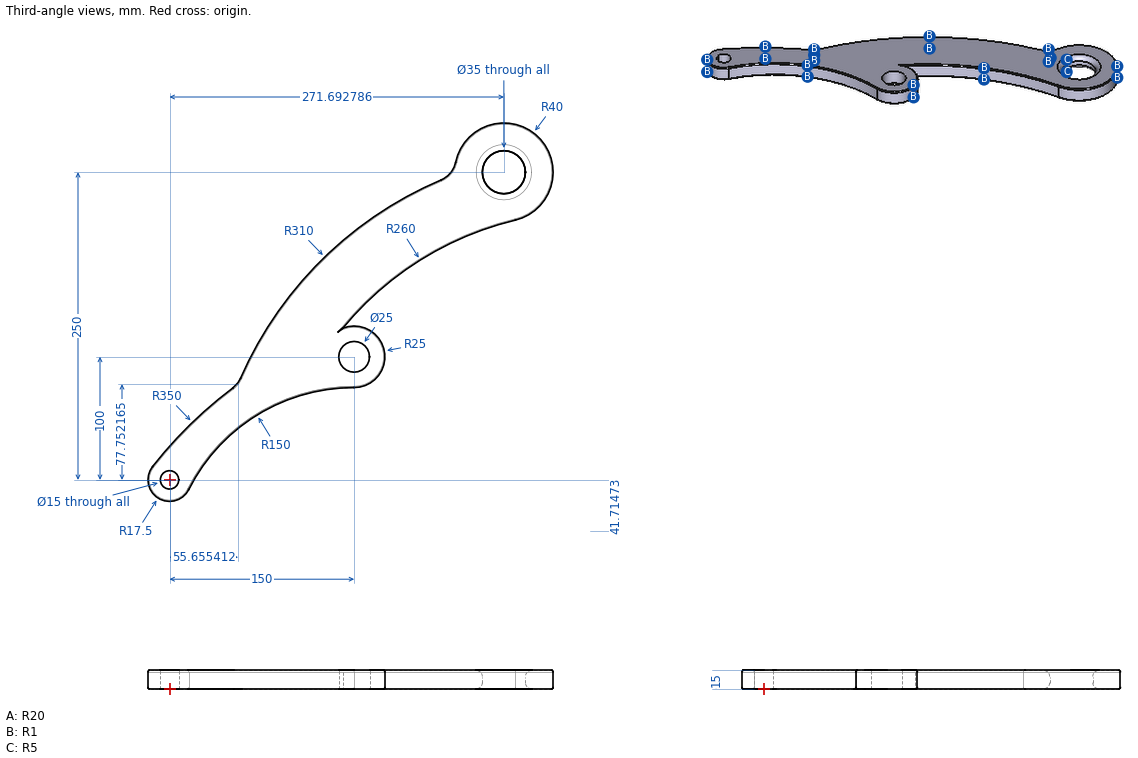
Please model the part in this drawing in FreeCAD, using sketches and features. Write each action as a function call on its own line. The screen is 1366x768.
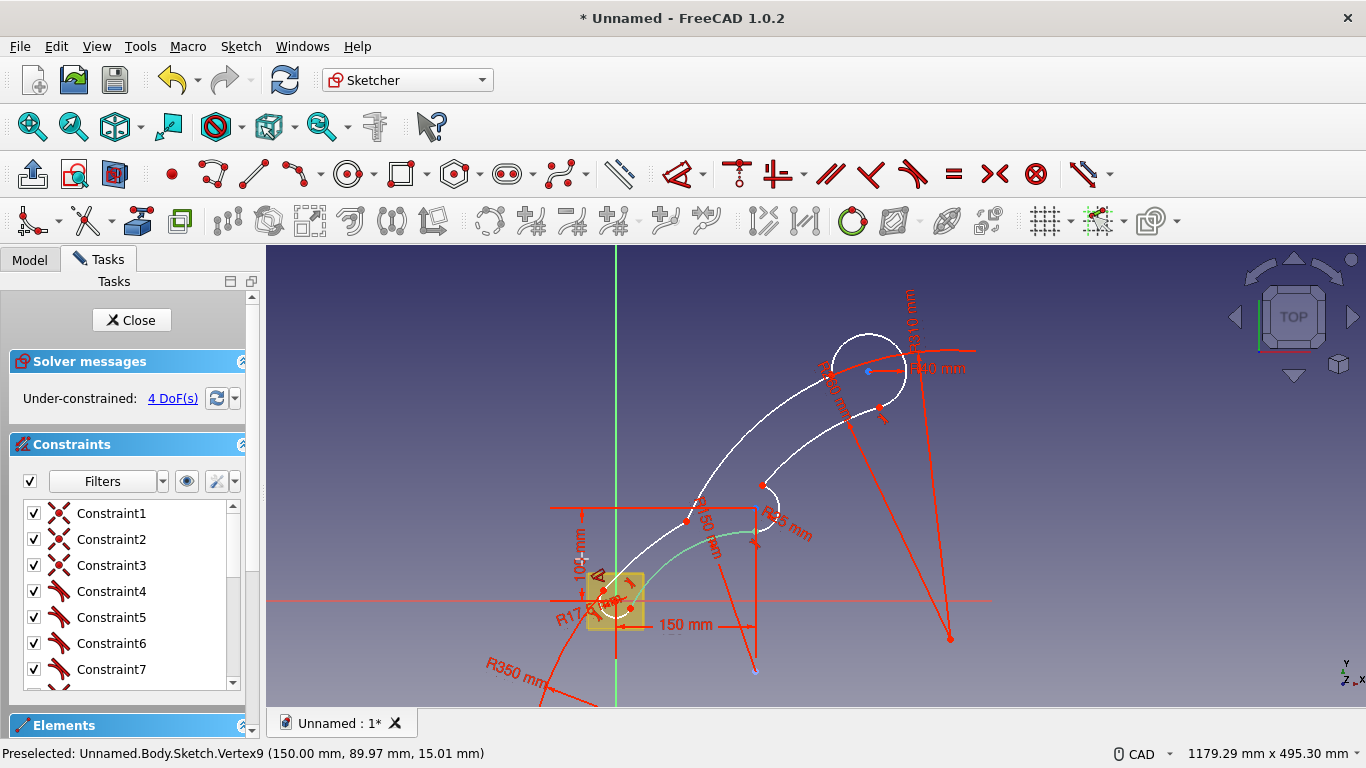
click(869, 372)
click(582, 486)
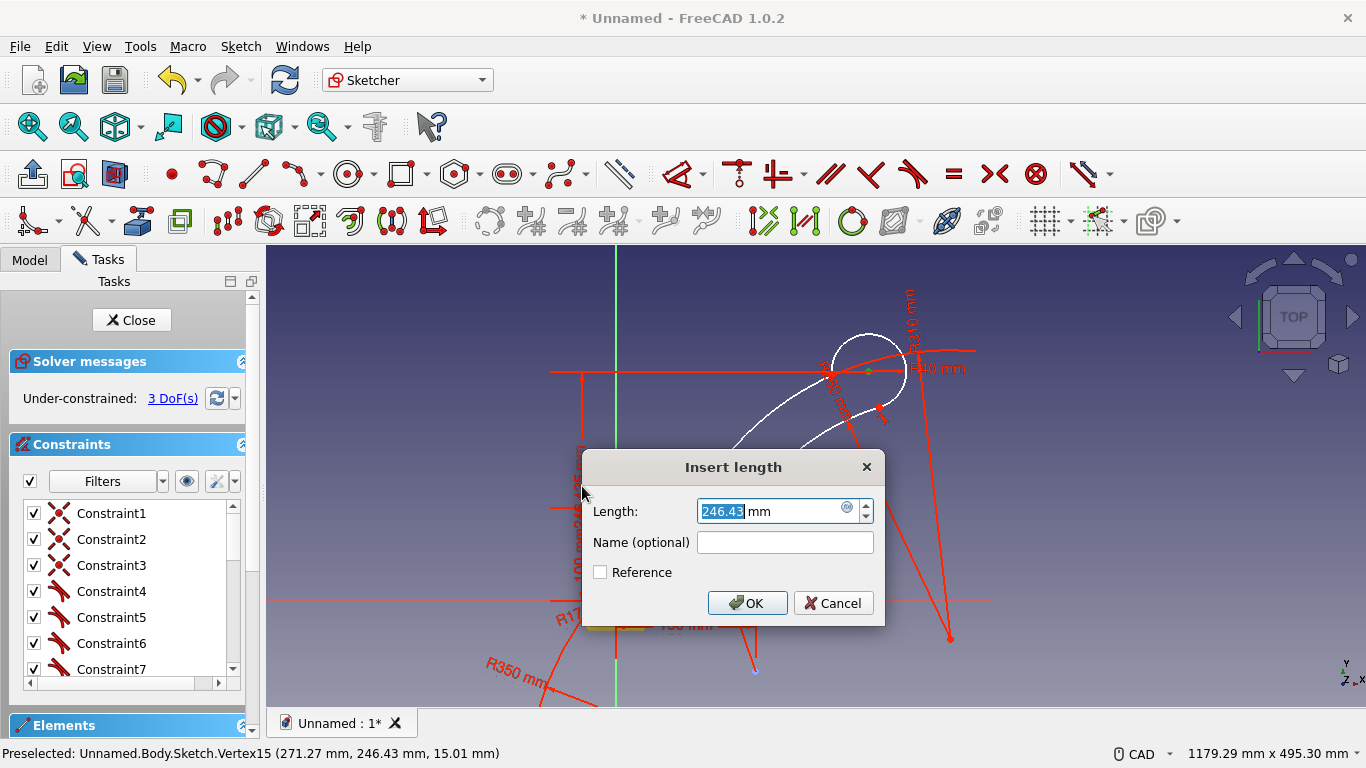
text(250)
key(Return)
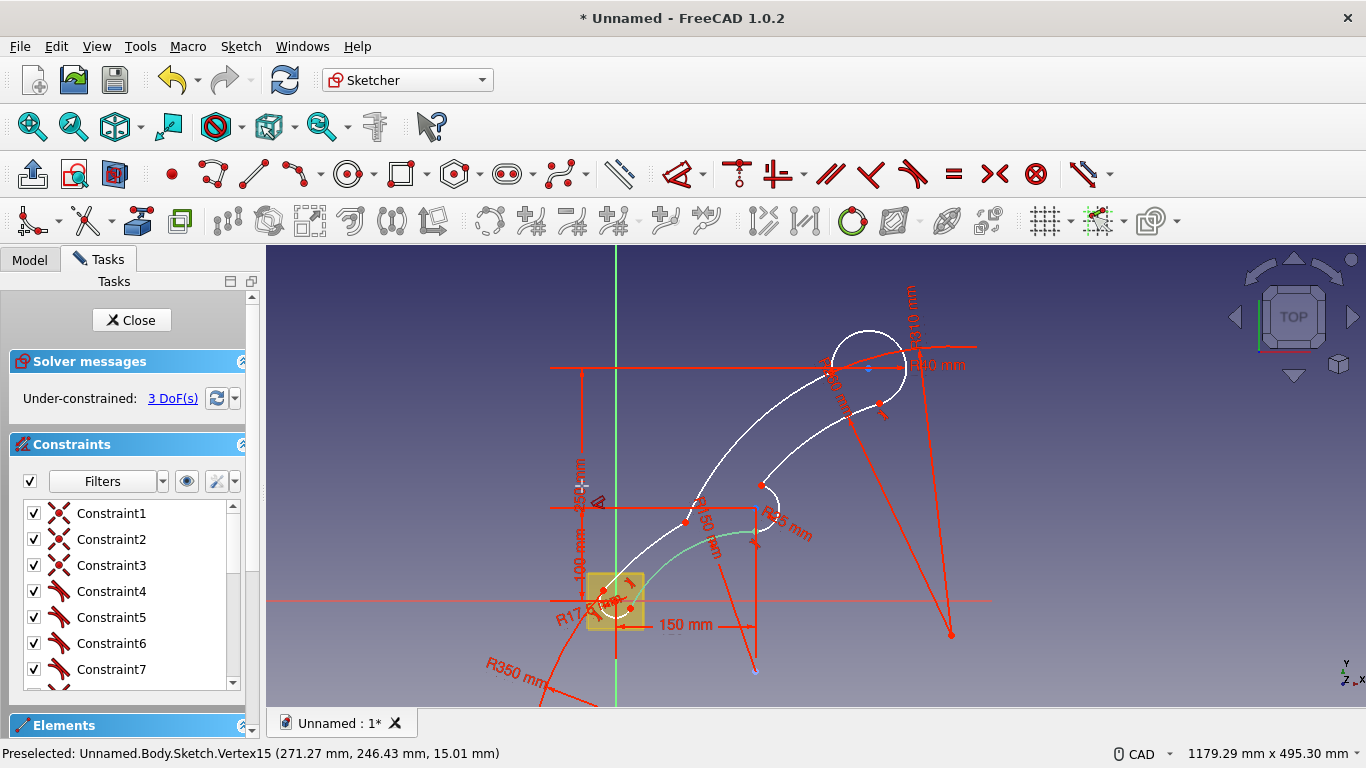
click(952, 636)
click(986, 618)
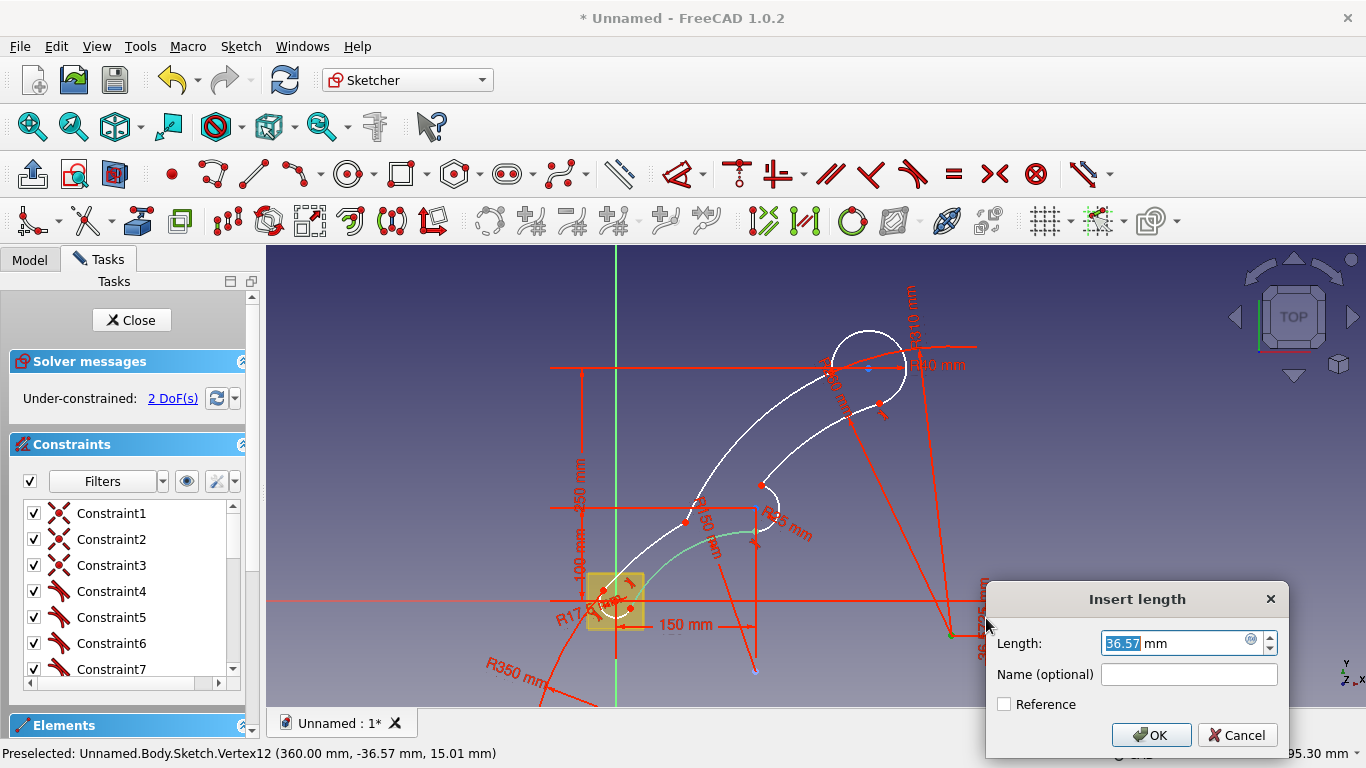
text(41.71473)
key(Return)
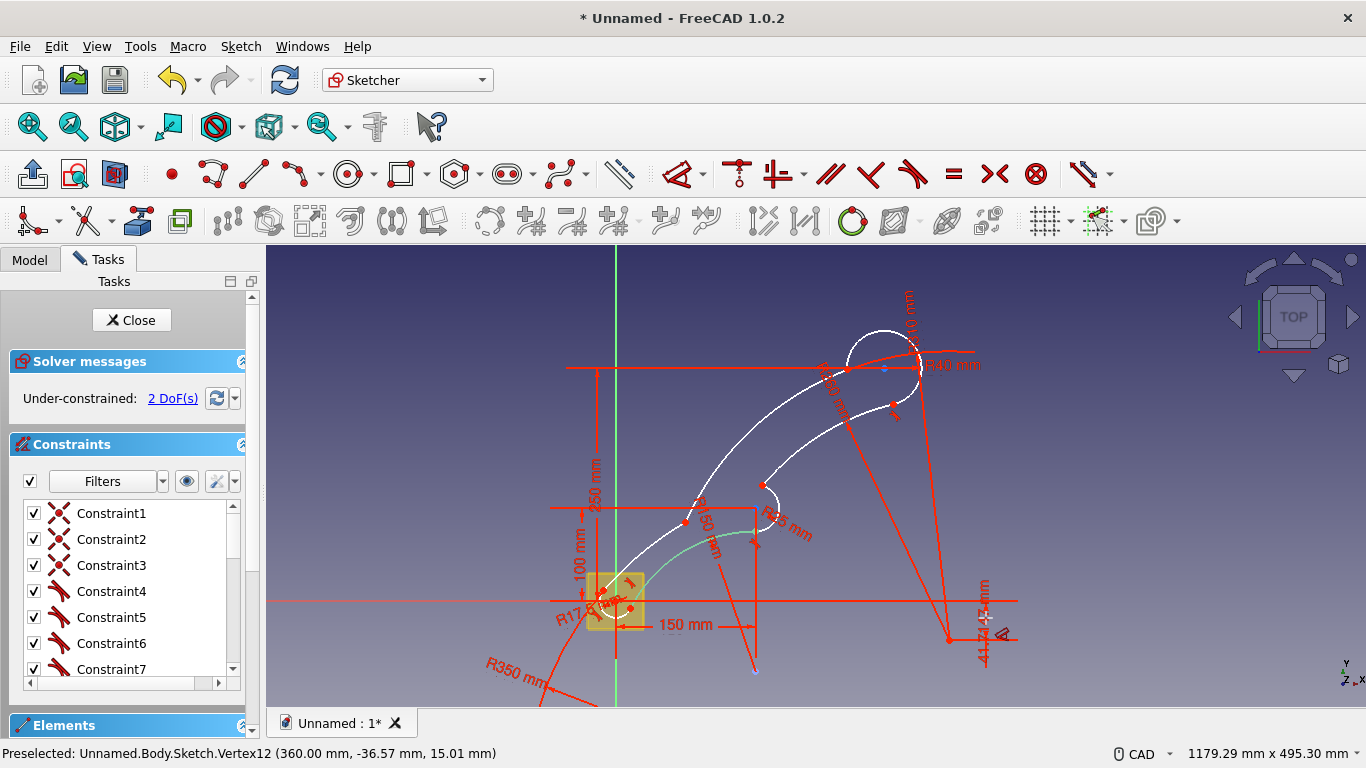
click(686, 522)
click(667, 488)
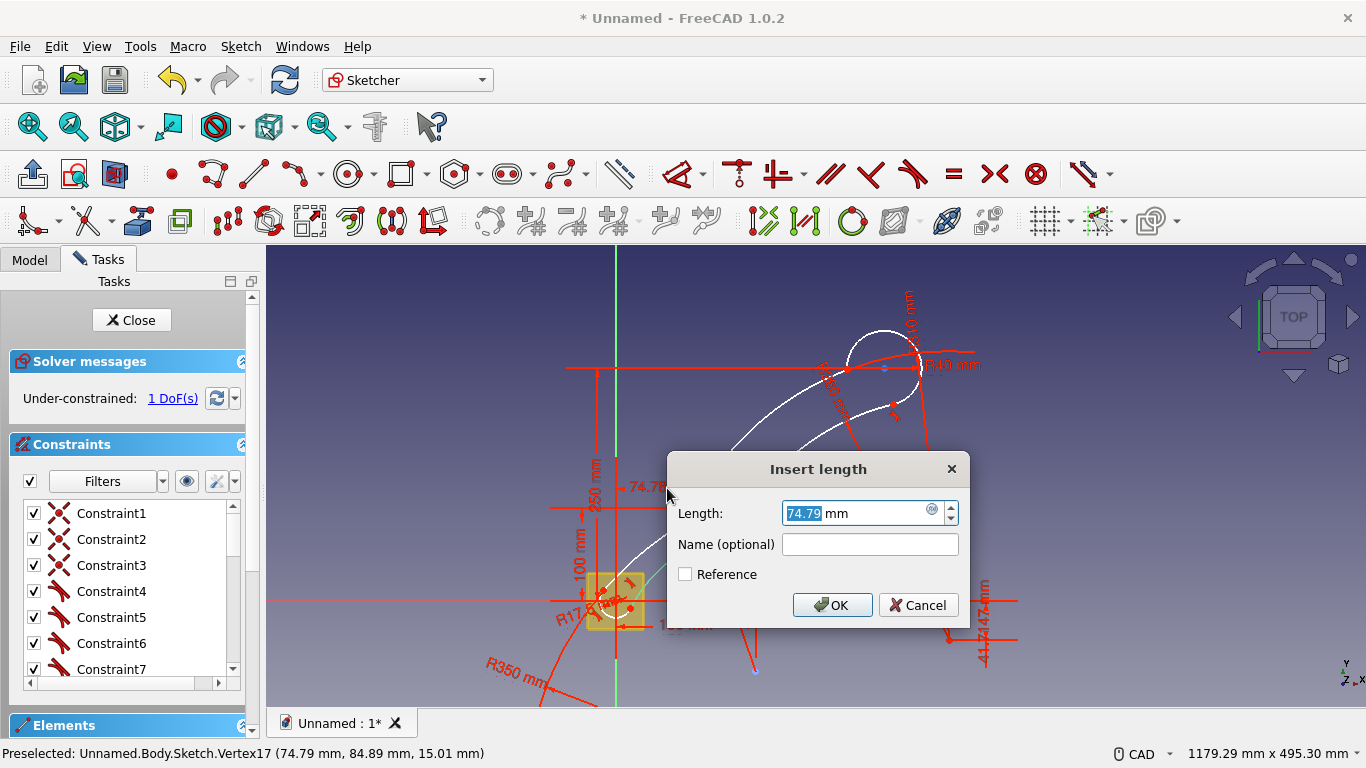
text(55.655412)
key(Return)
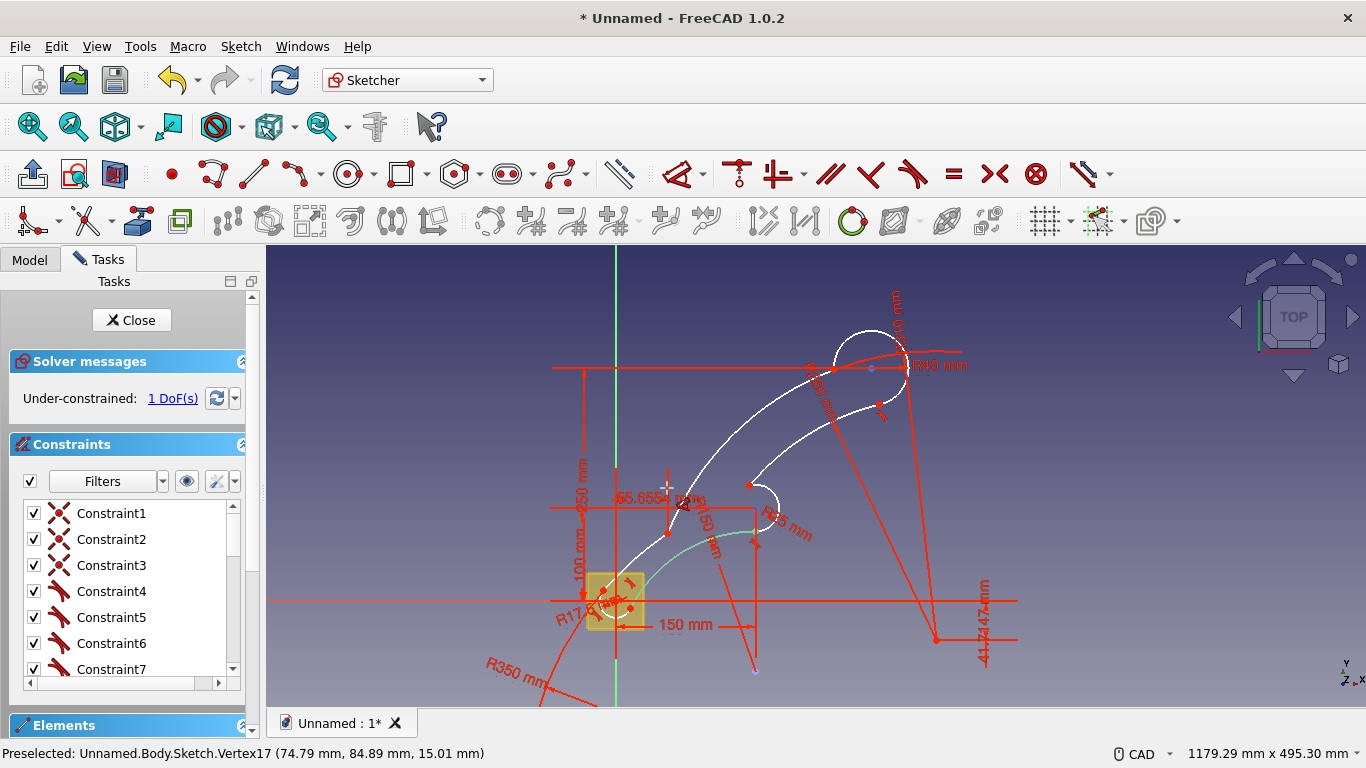
click(668, 533)
click(582, 583)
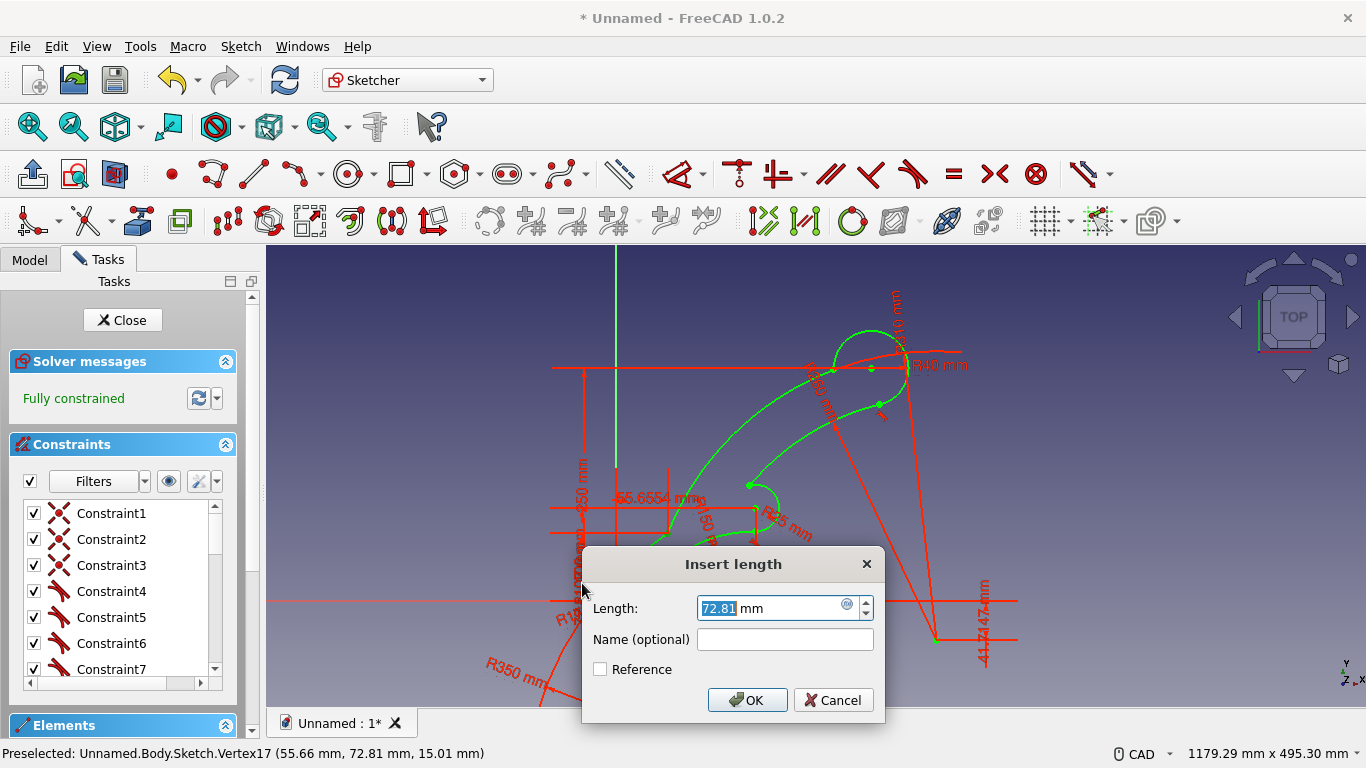
text(77.752165)
key(Return)
key(Escape)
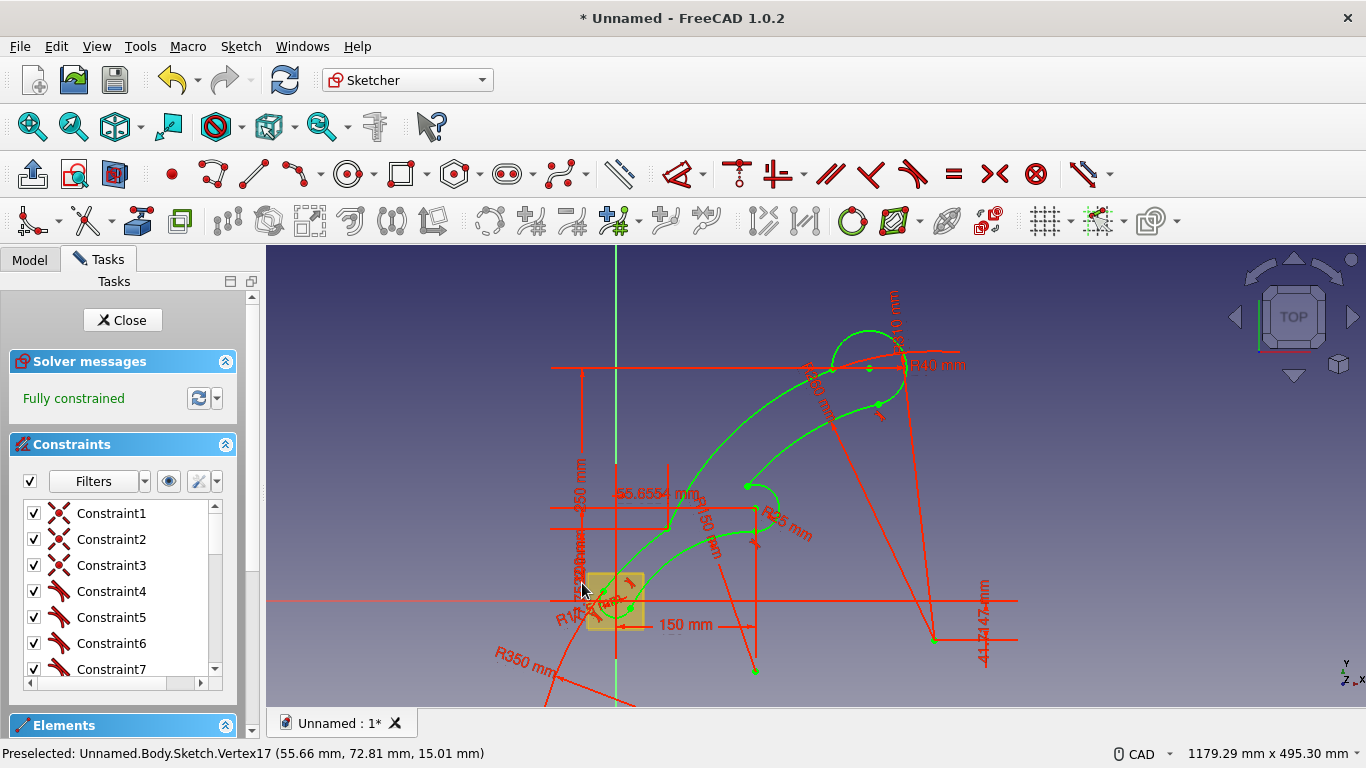
click(123, 320)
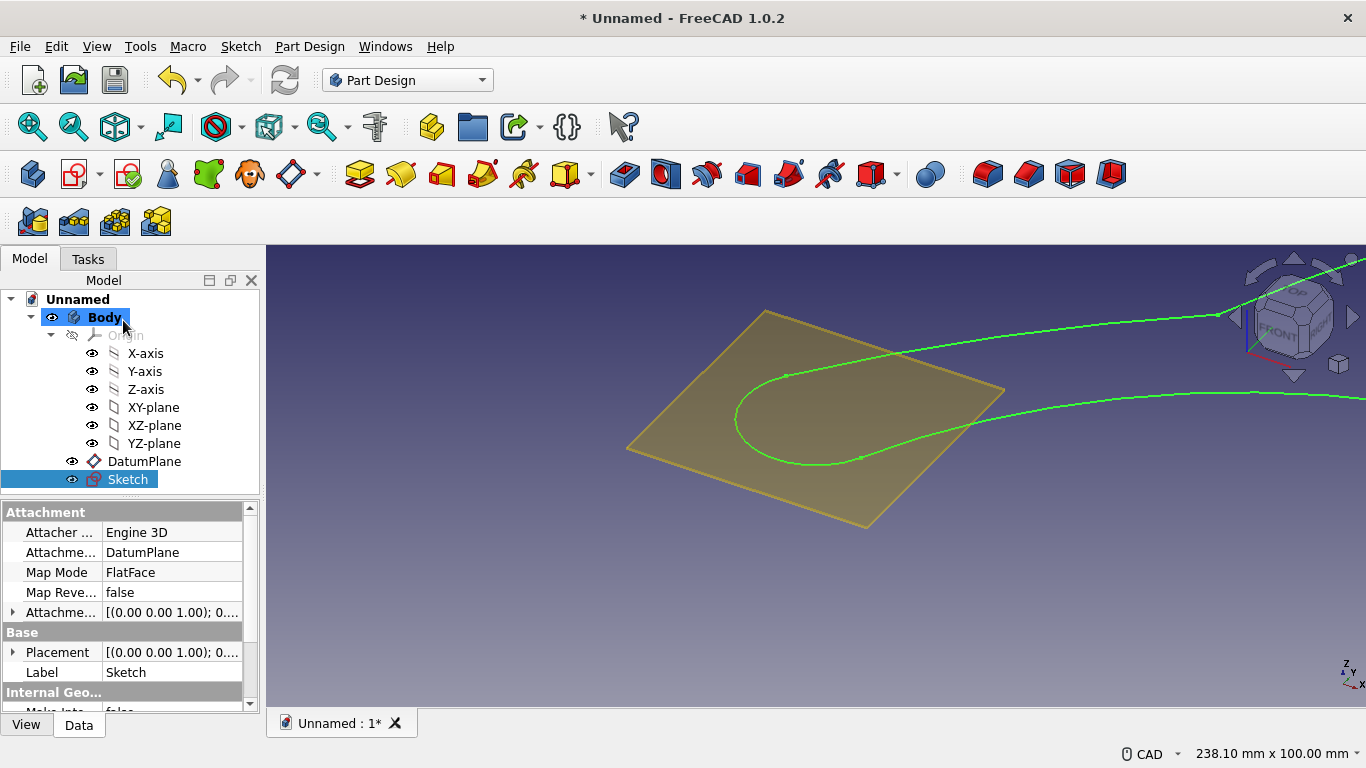
click(360, 174)